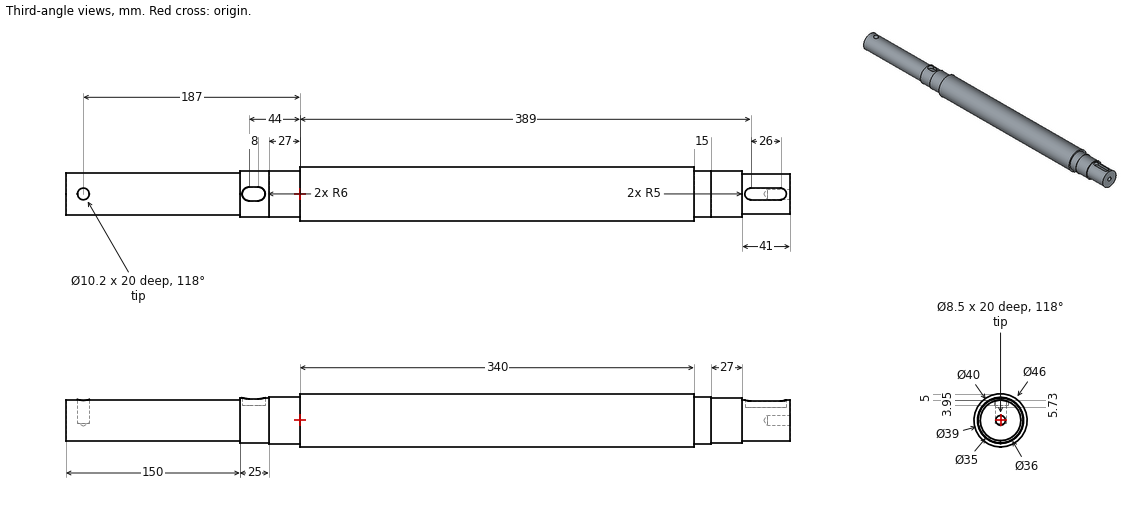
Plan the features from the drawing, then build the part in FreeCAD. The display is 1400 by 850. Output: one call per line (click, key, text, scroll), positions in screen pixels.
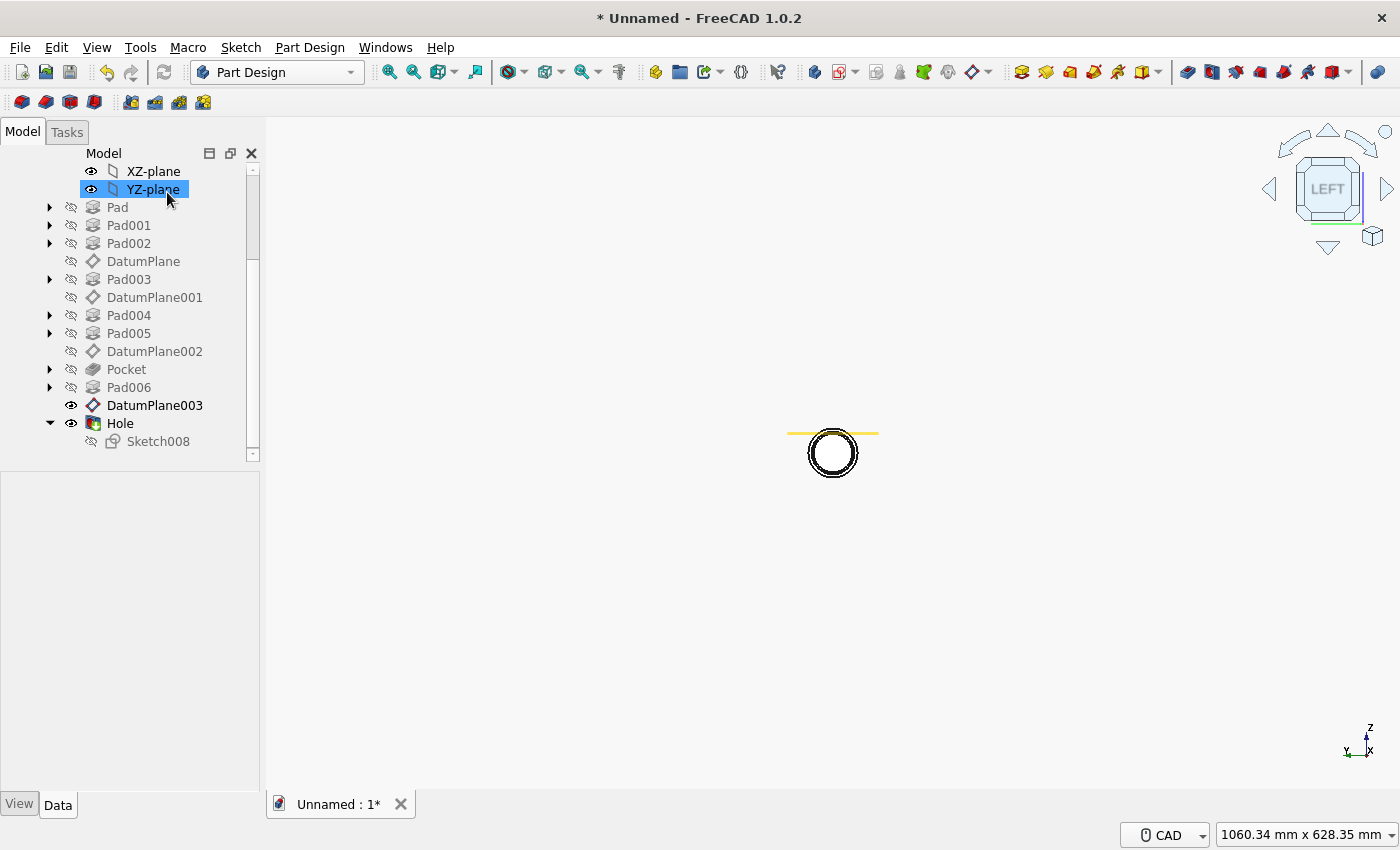
click(116, 405)
key(space)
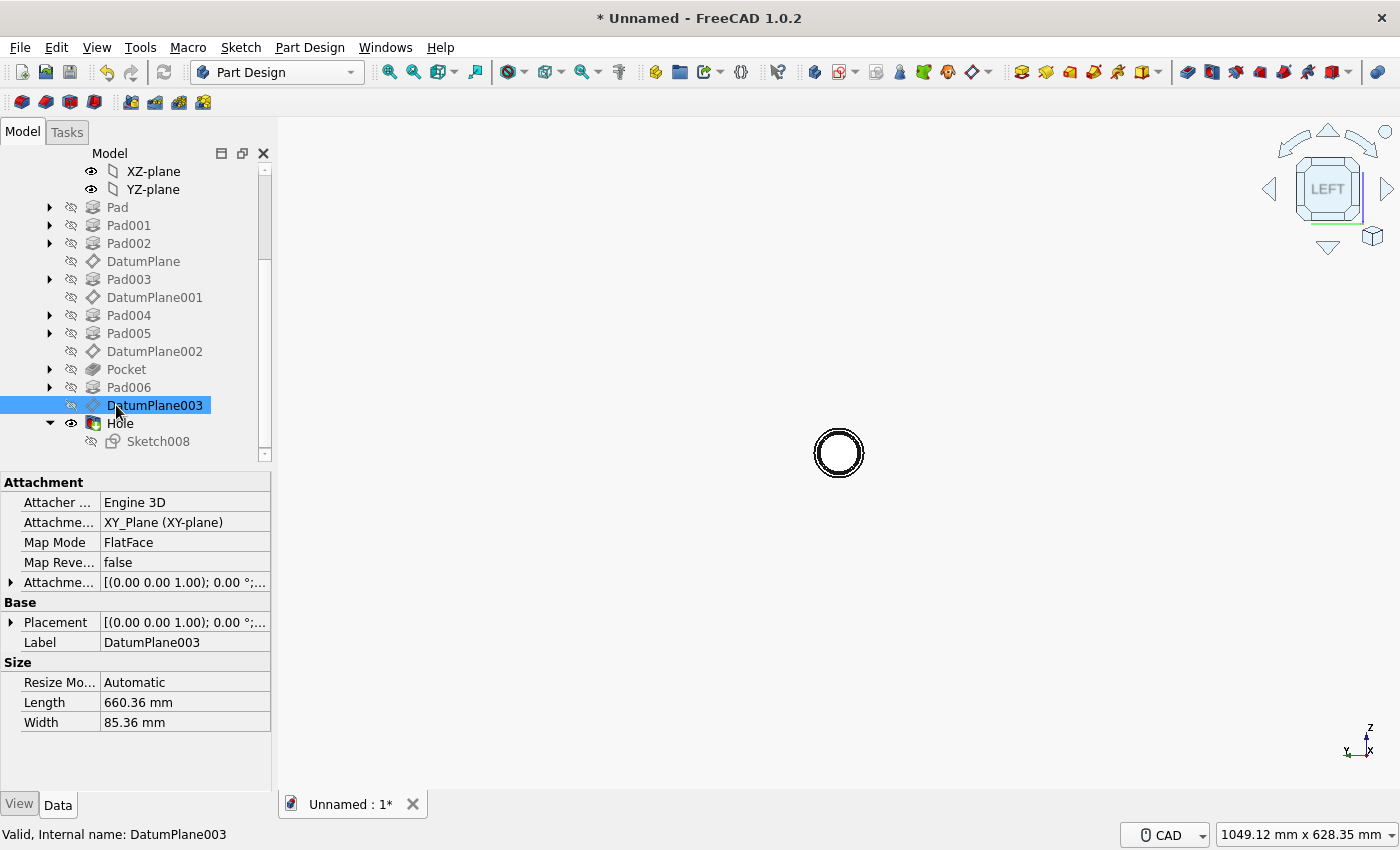
click(390, 72)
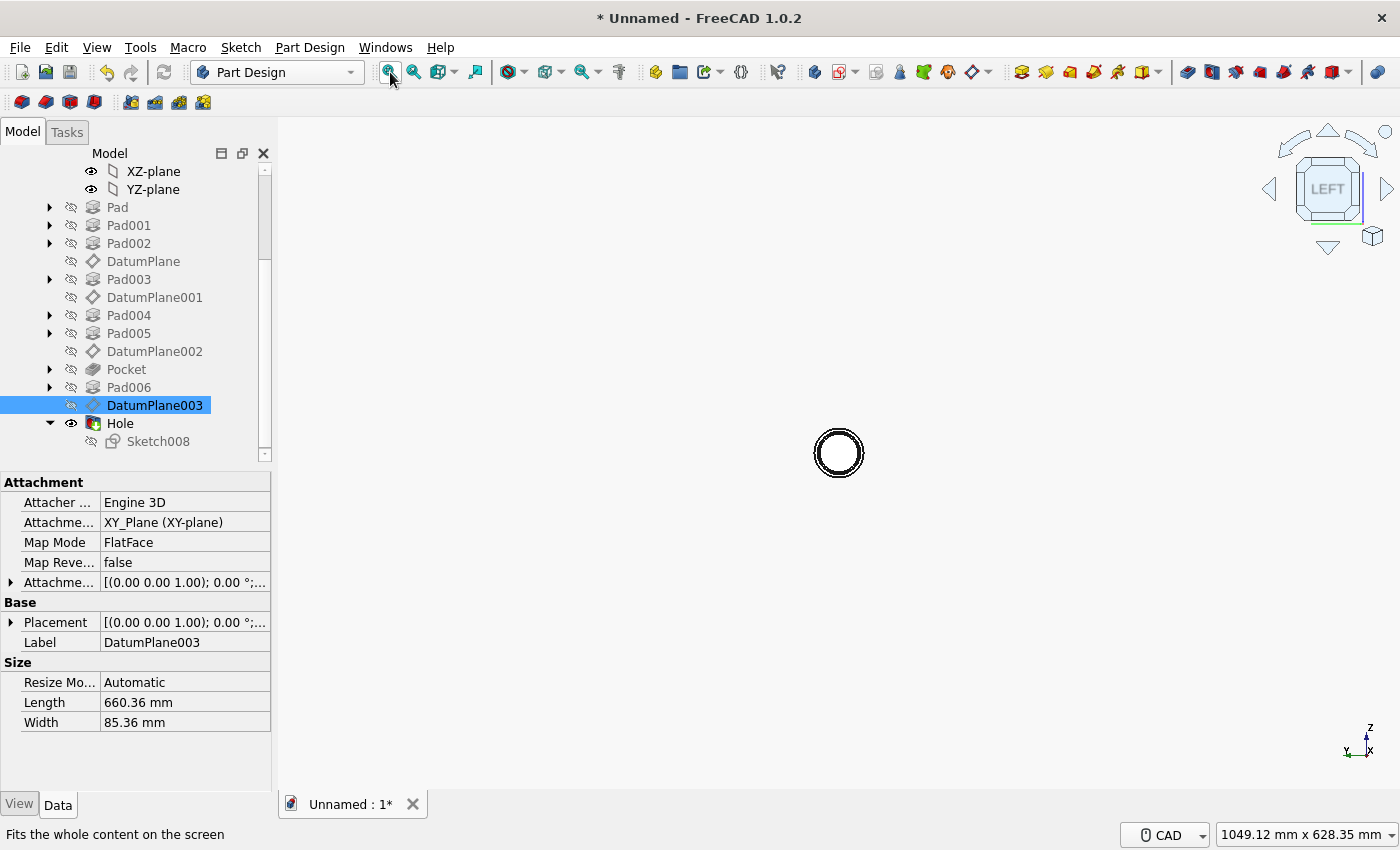
key(0)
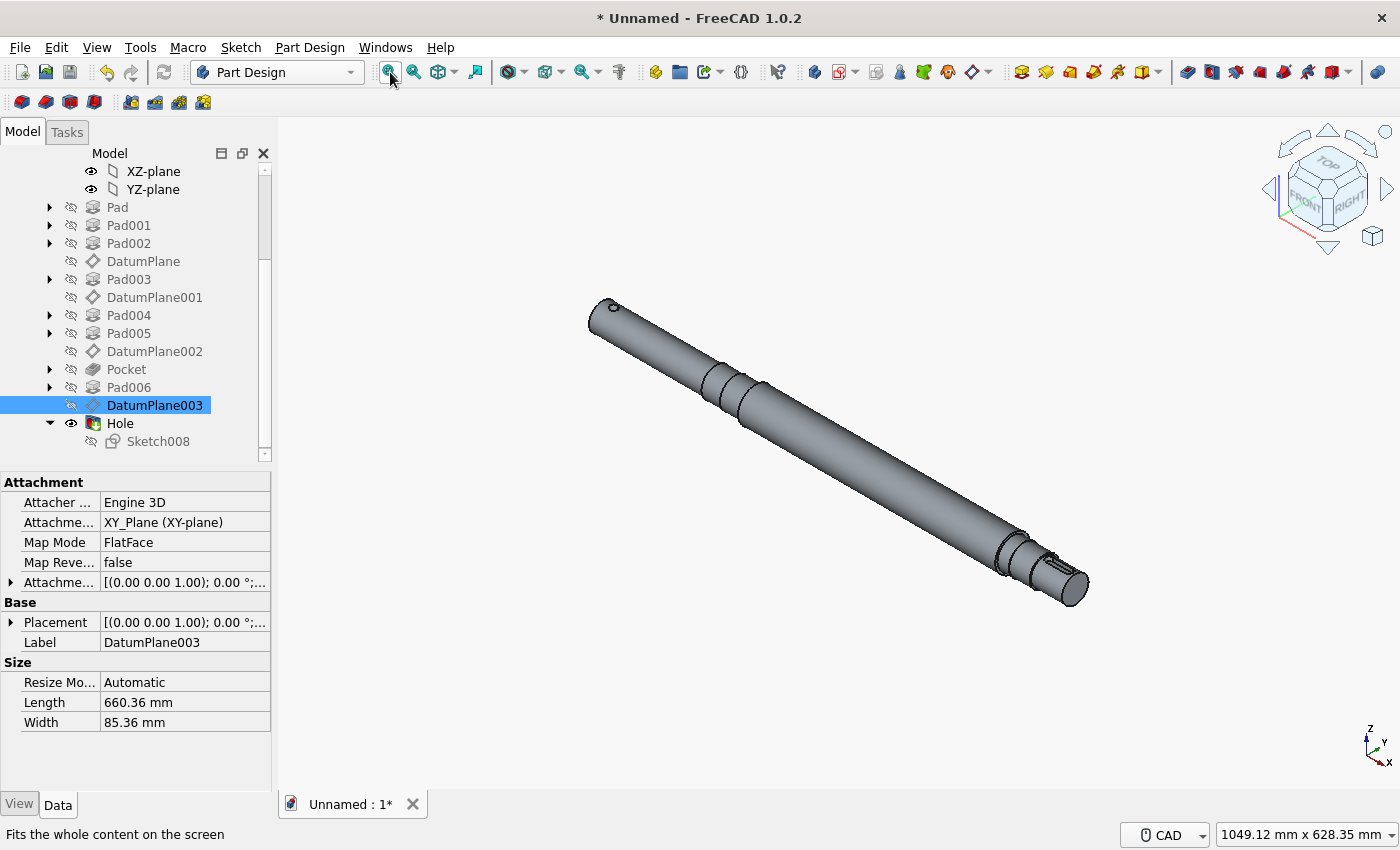
click(1075, 588)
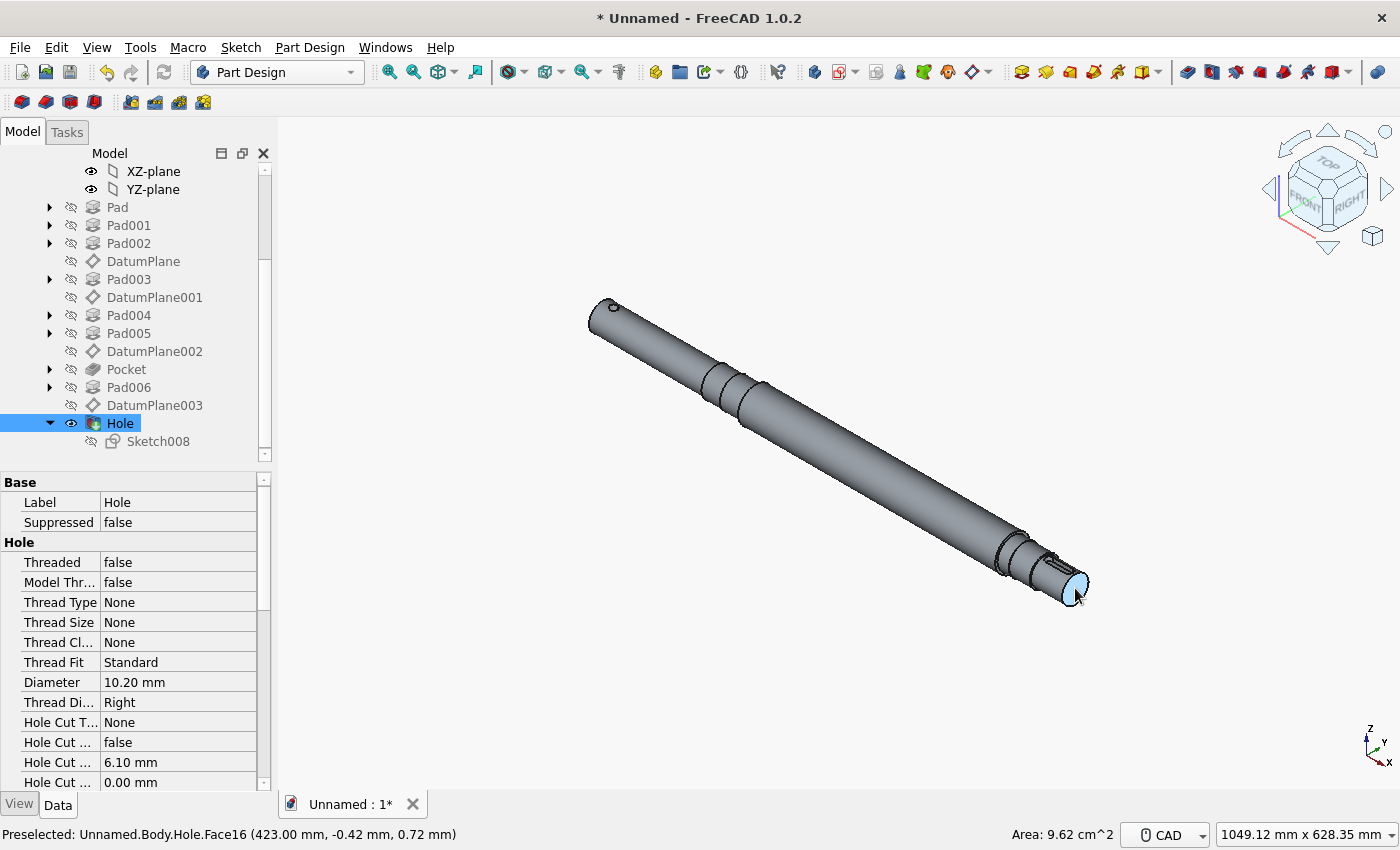
click(840, 72)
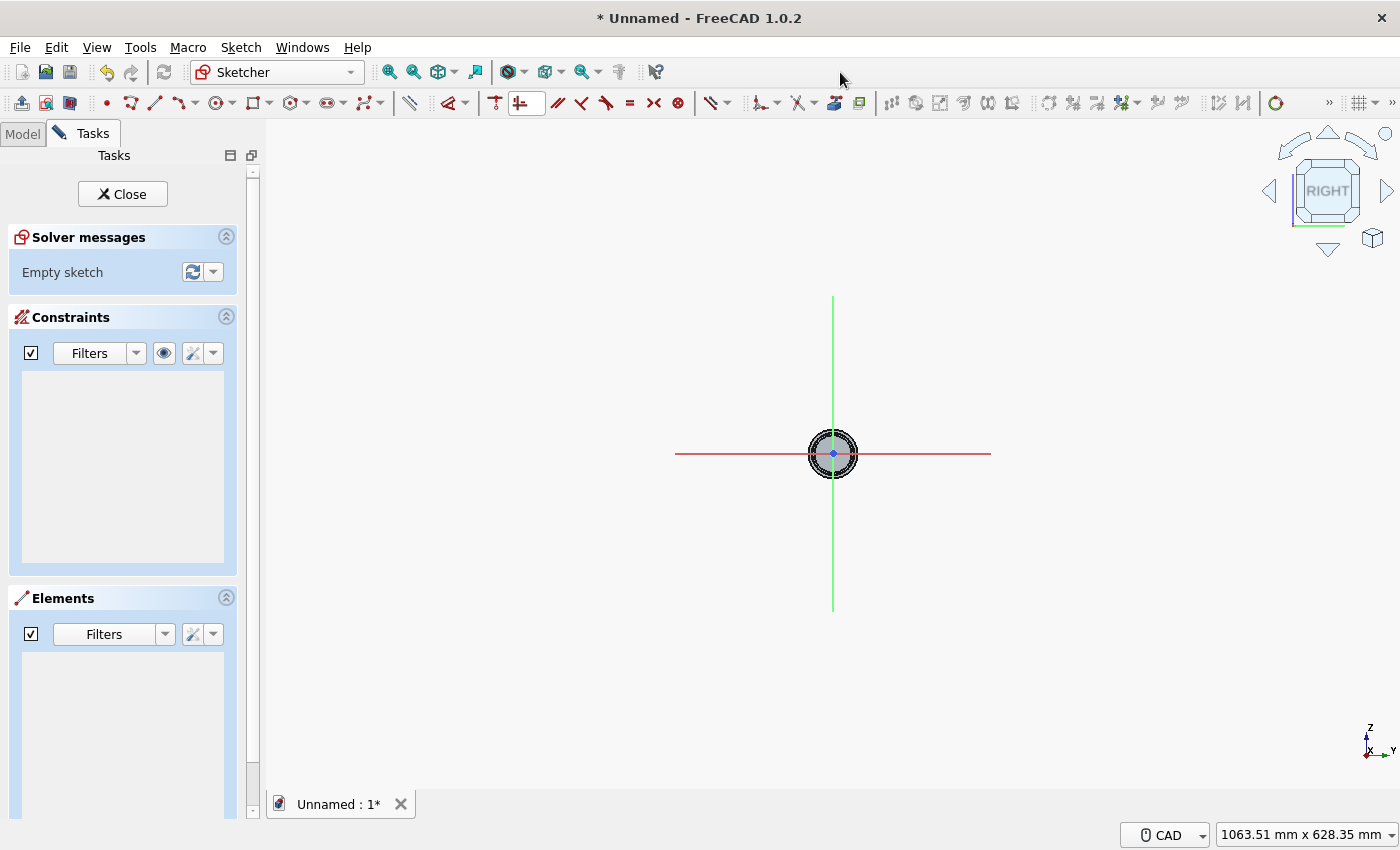
scroll(837, 454, up, 15)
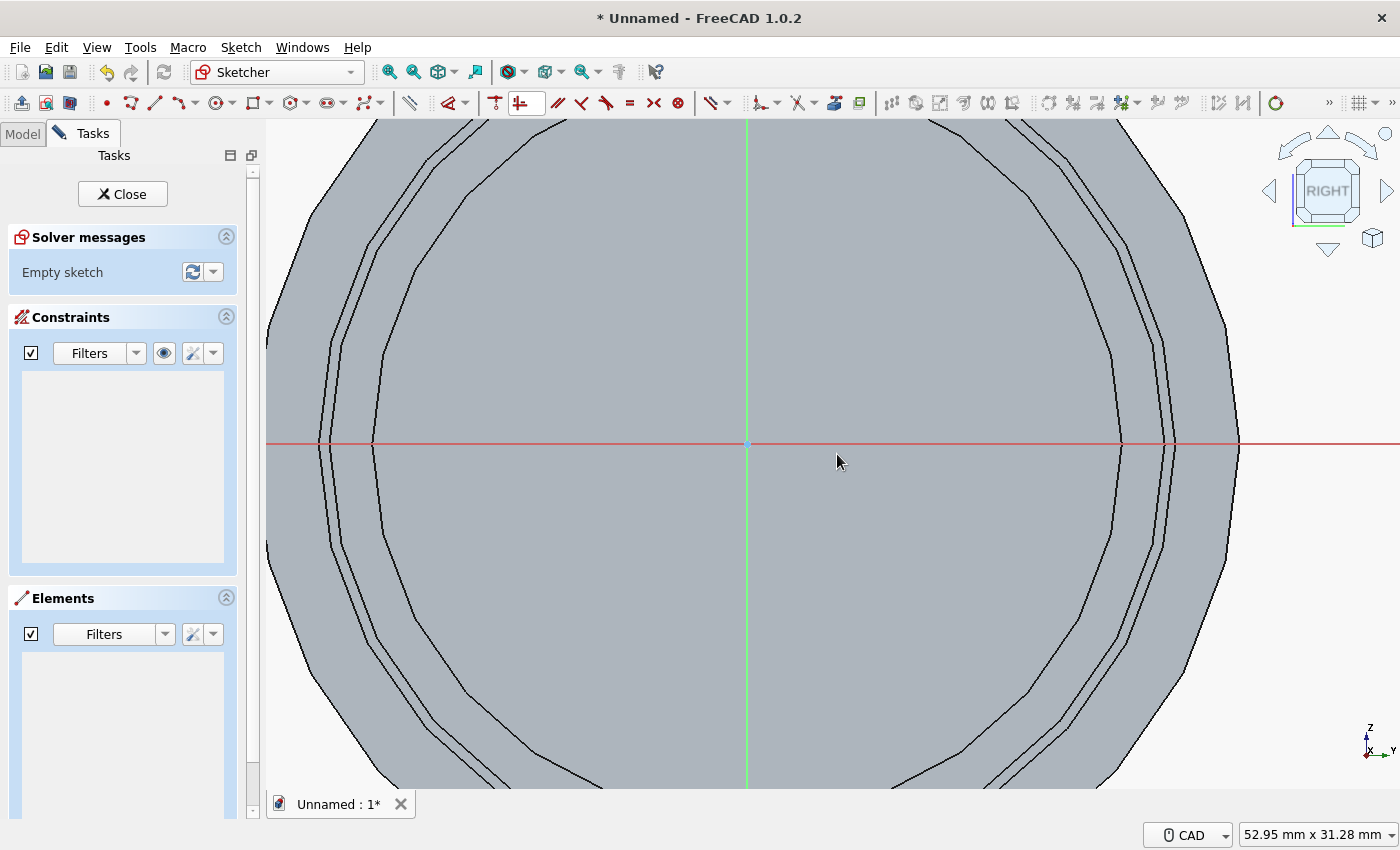
scroll(733, 437, up, 4)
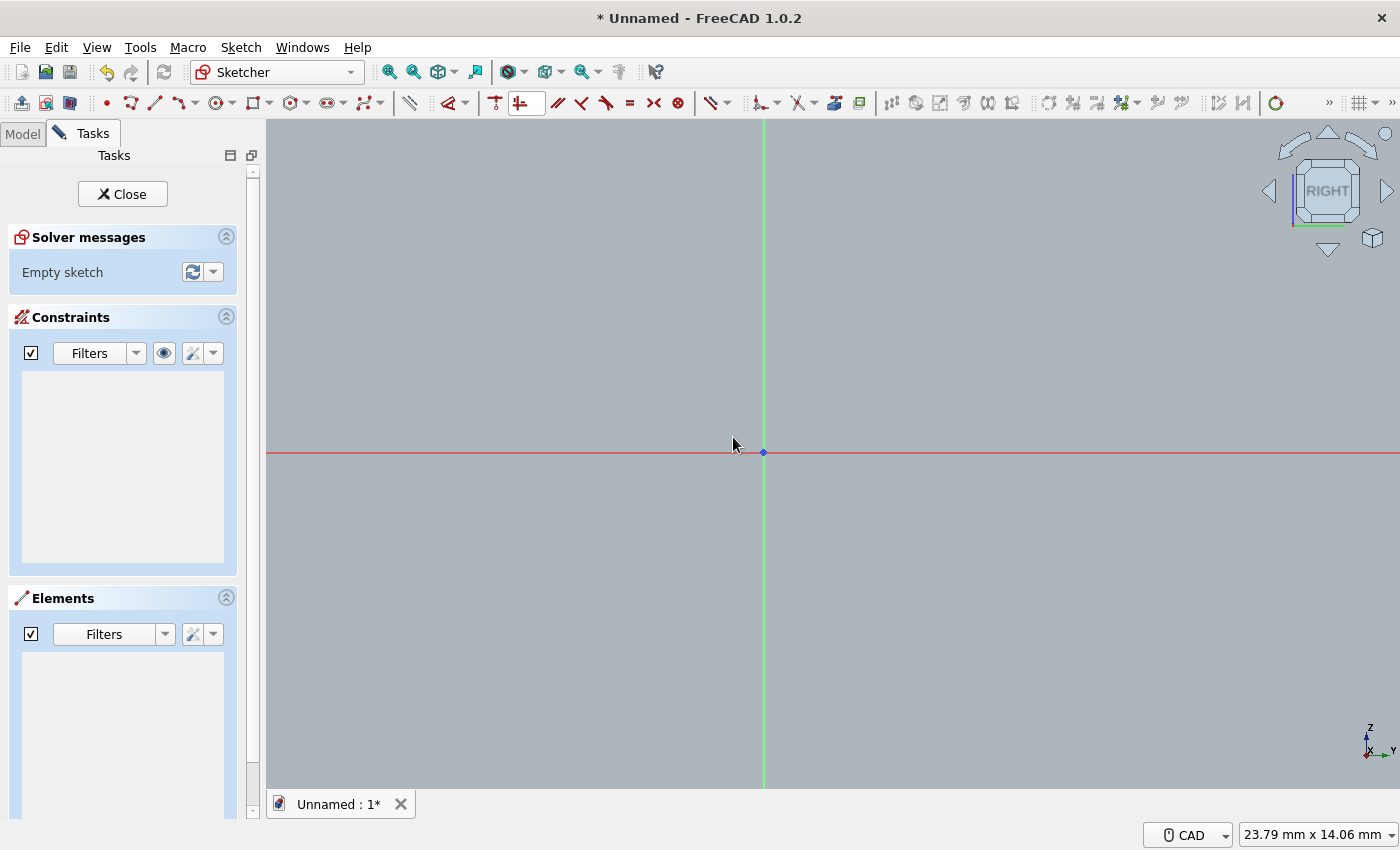
key(g)
key(c)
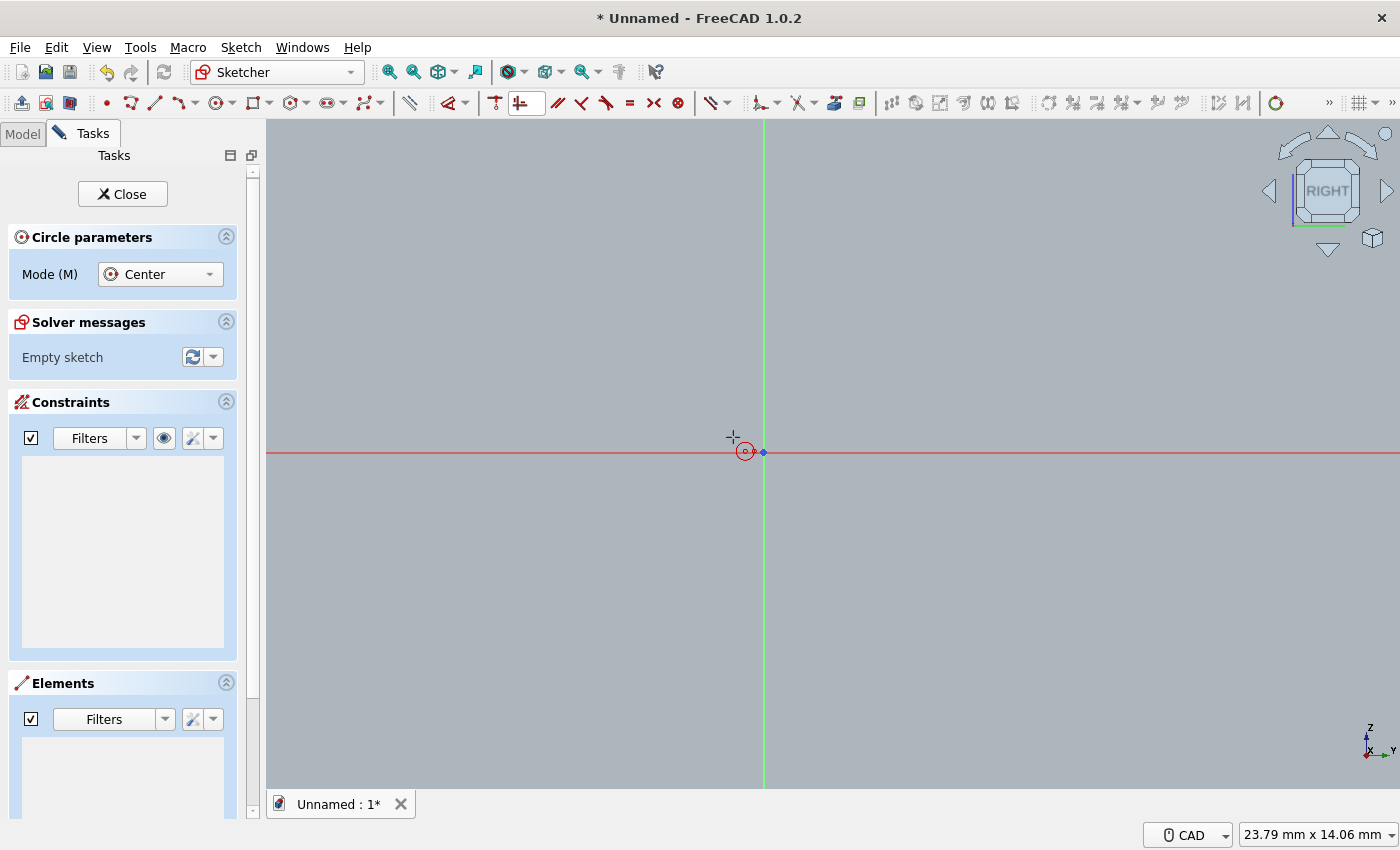
click(764, 453)
click(907, 310)
key(Escape)